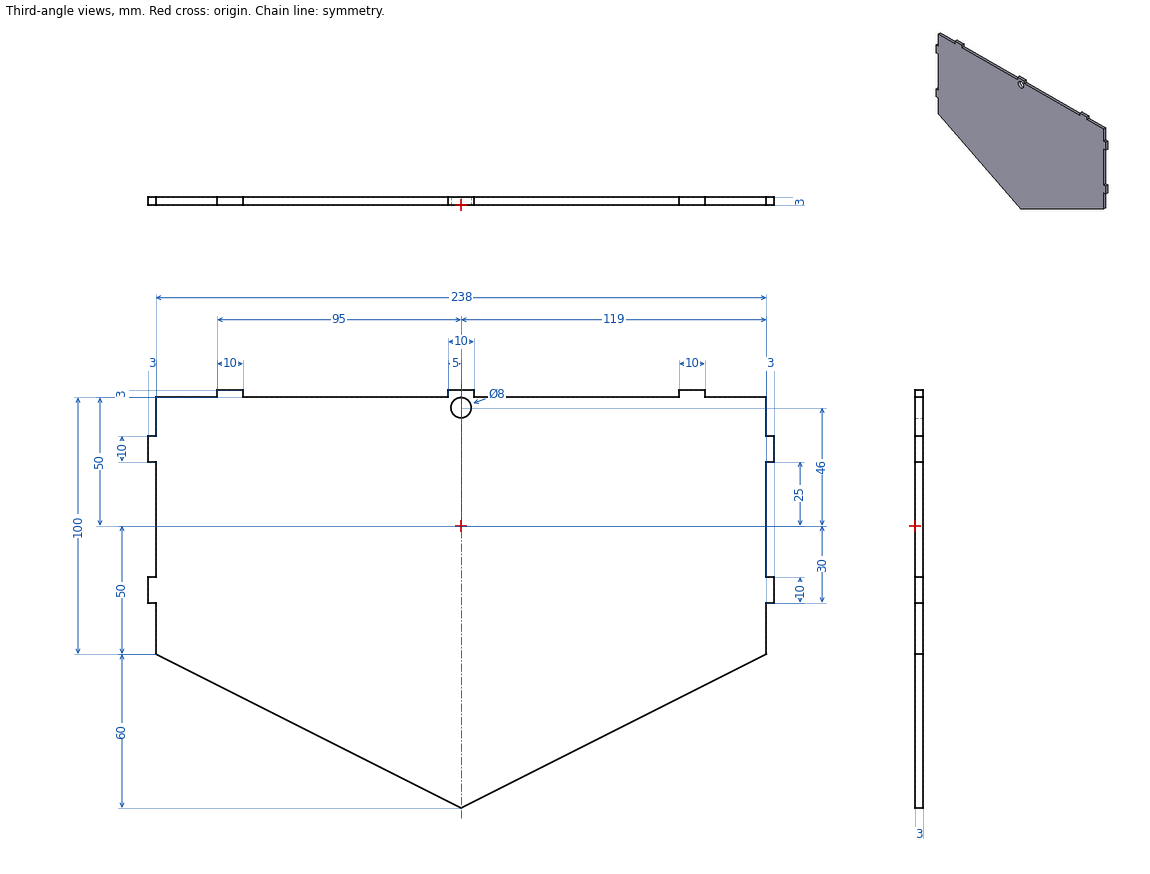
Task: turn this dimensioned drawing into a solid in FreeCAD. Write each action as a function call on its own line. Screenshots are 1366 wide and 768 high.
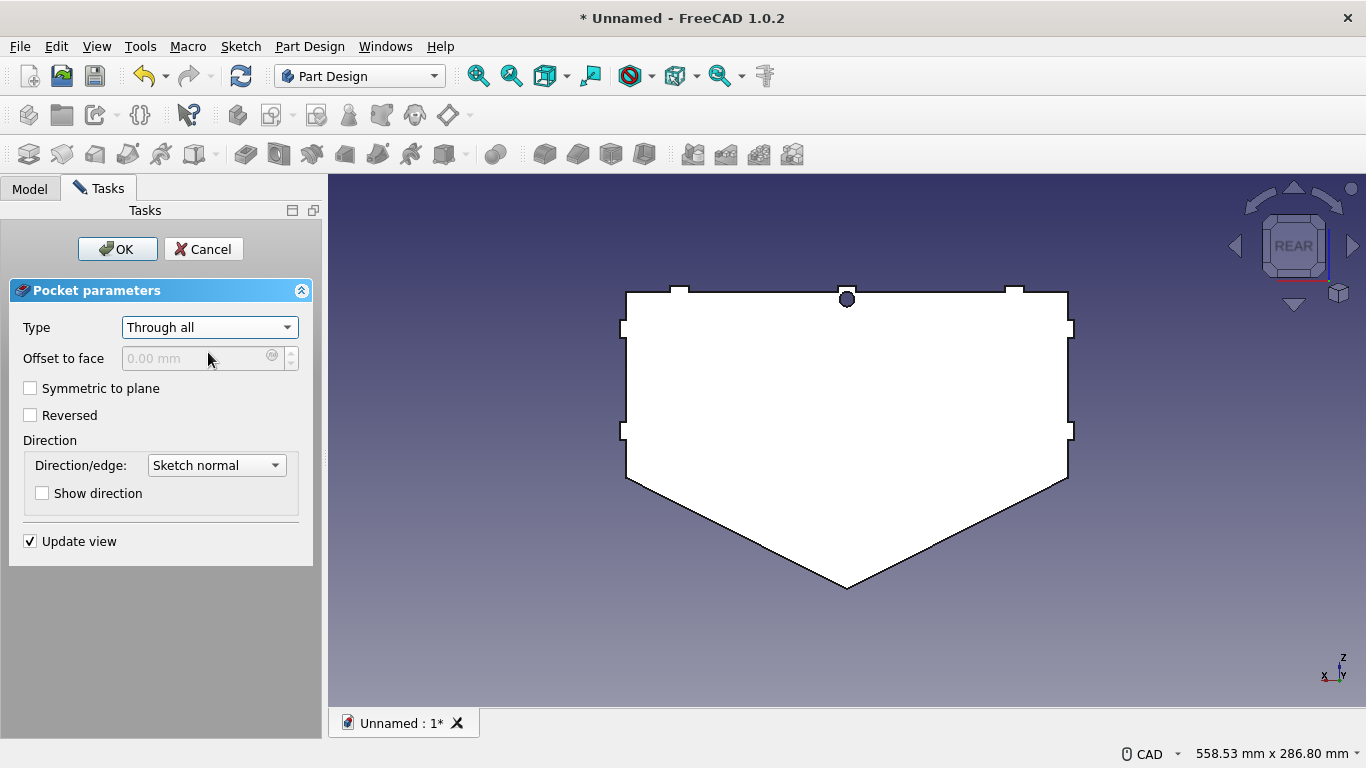
click(118, 249)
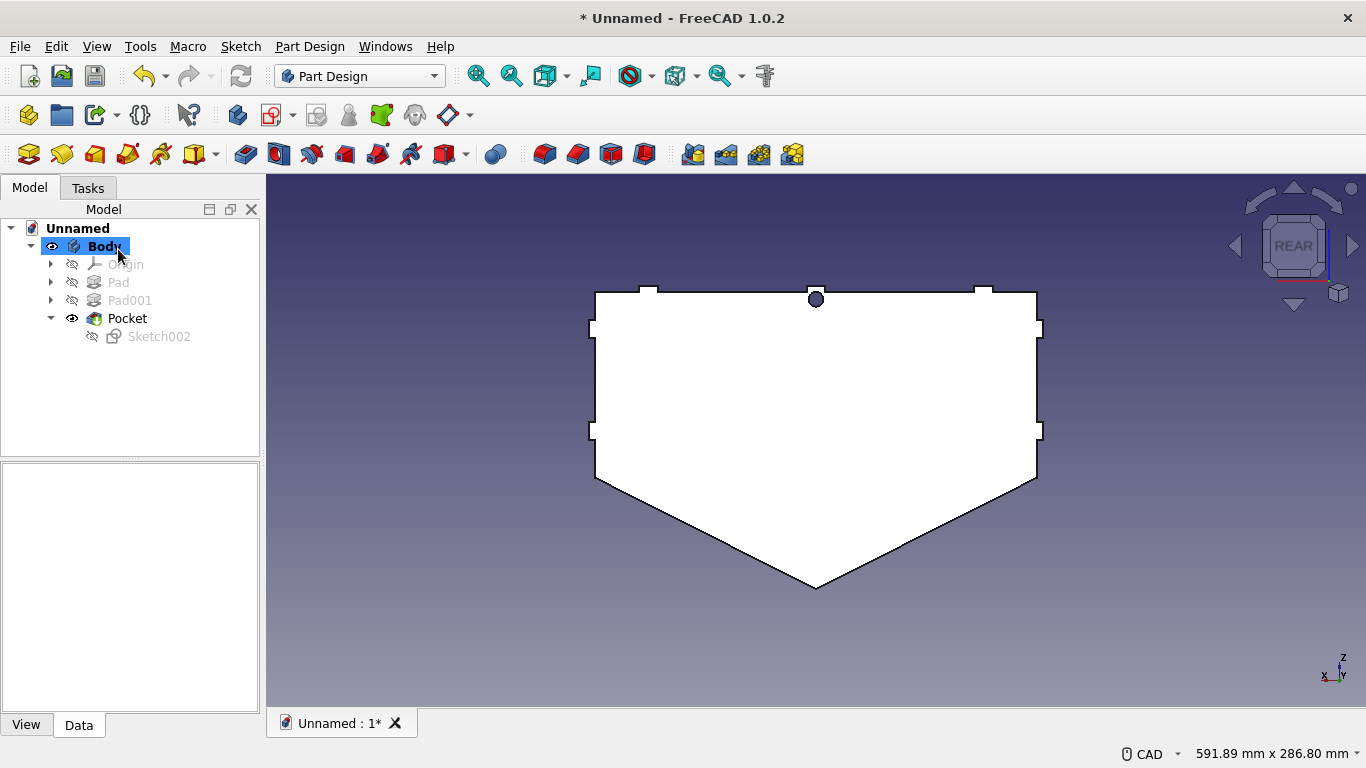
key(0)